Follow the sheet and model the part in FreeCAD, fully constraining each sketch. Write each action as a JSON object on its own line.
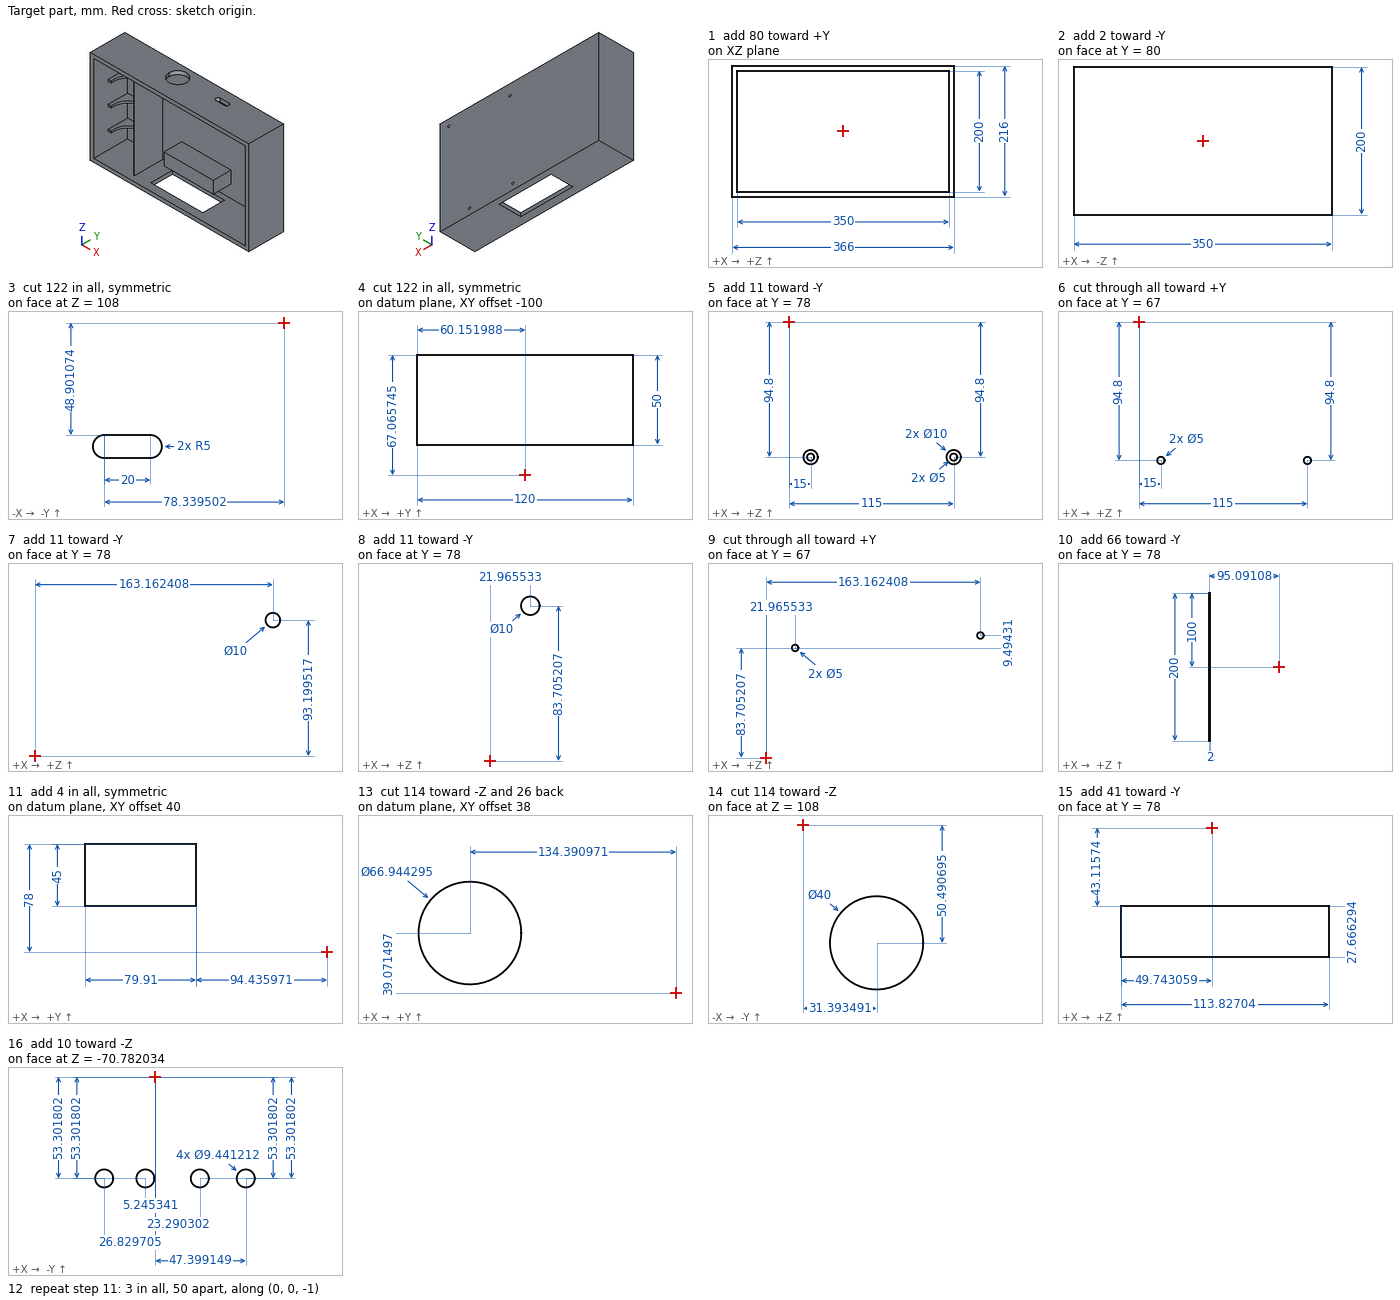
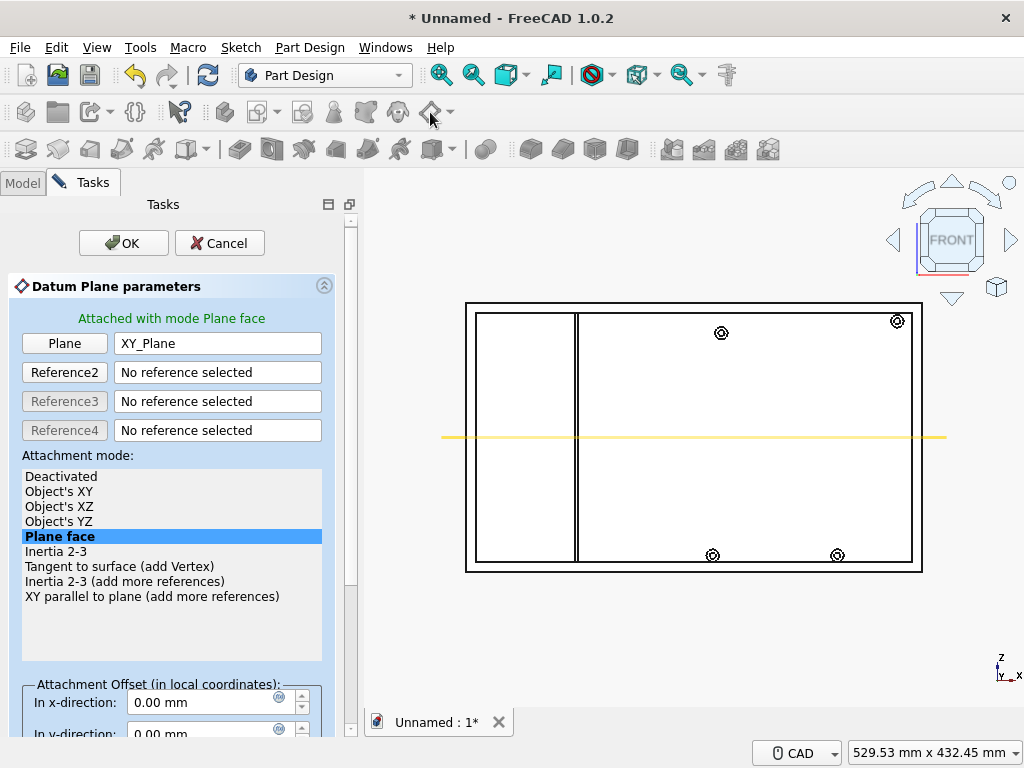
{"action": "scroll", "coordinate": [351, 475], "scroll_direction": "down", "scroll_amount": 2}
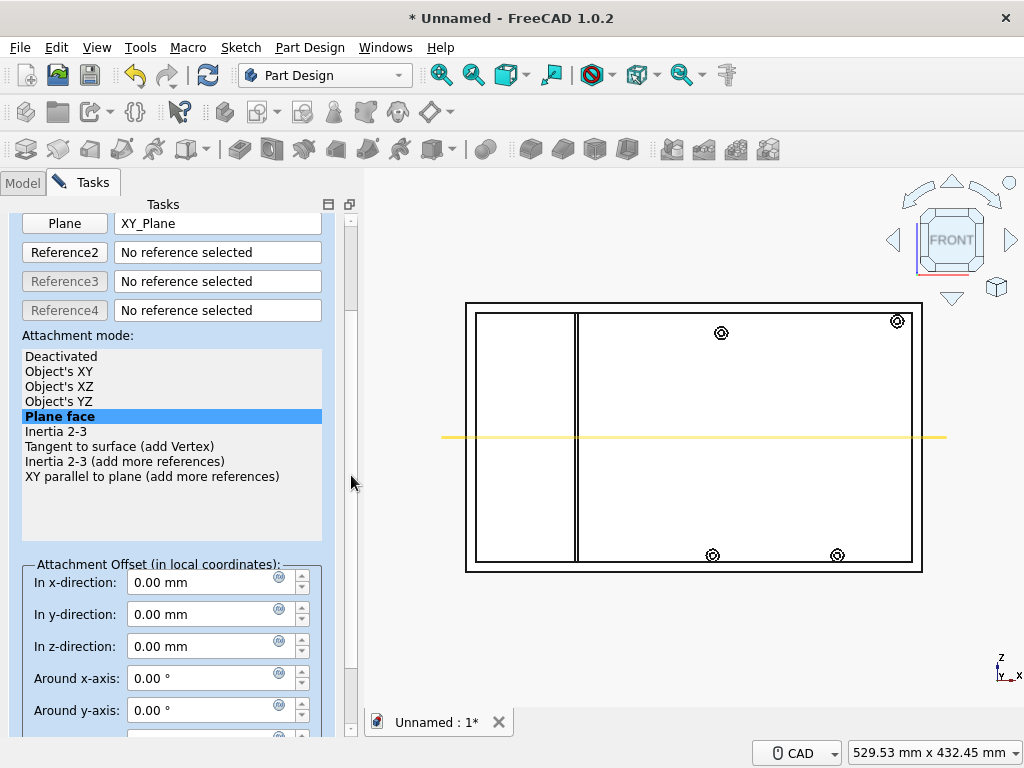
{"action": "triple_click", "coordinate": [210, 646]}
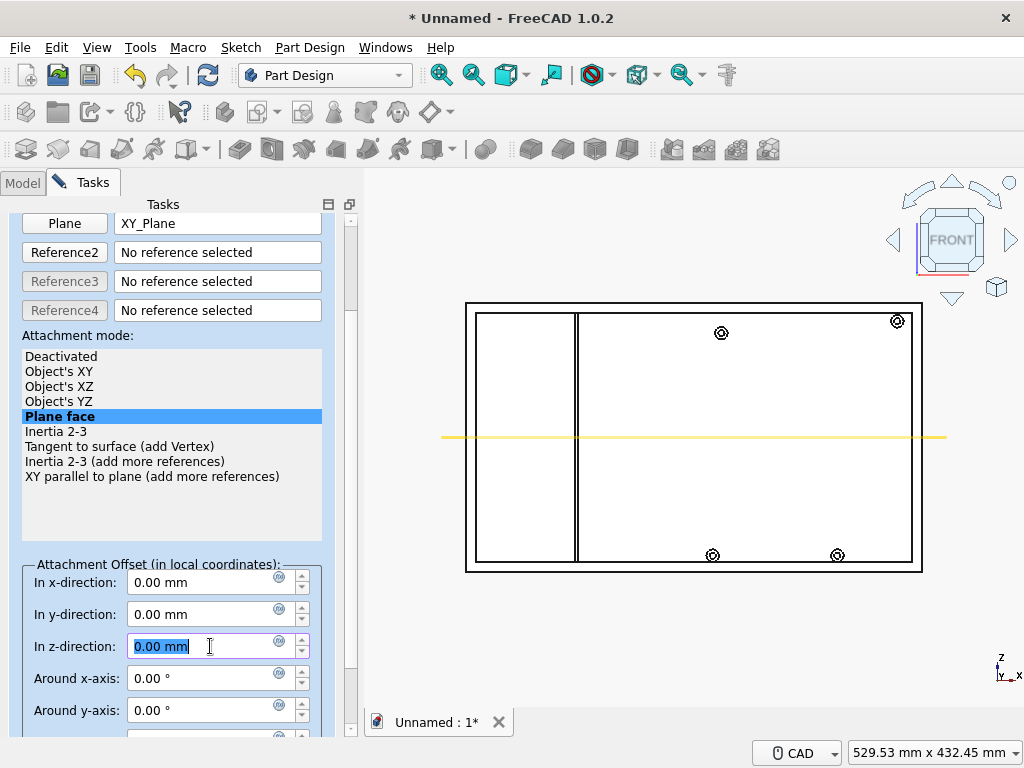
{"action": "type", "text": "40"}
{"action": "key", "text": "Tab"}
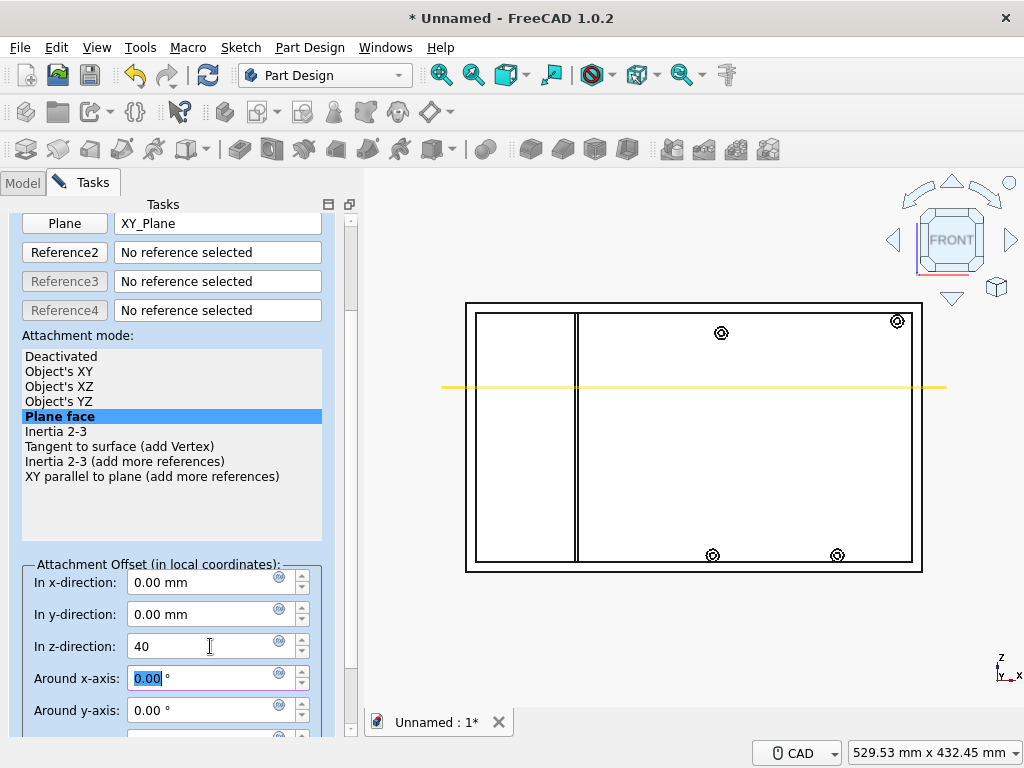
{"action": "scroll", "coordinate": [351, 475], "scroll_direction": "up", "scroll_amount": 3}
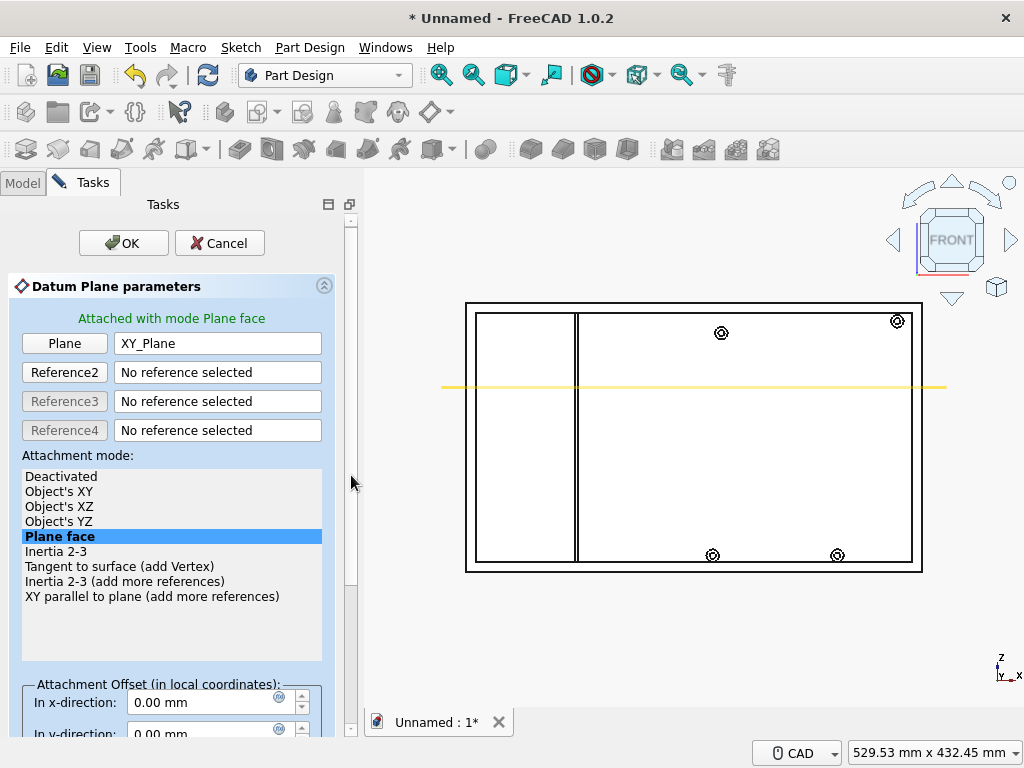
{"action": "left_click", "coordinate": [124, 243]}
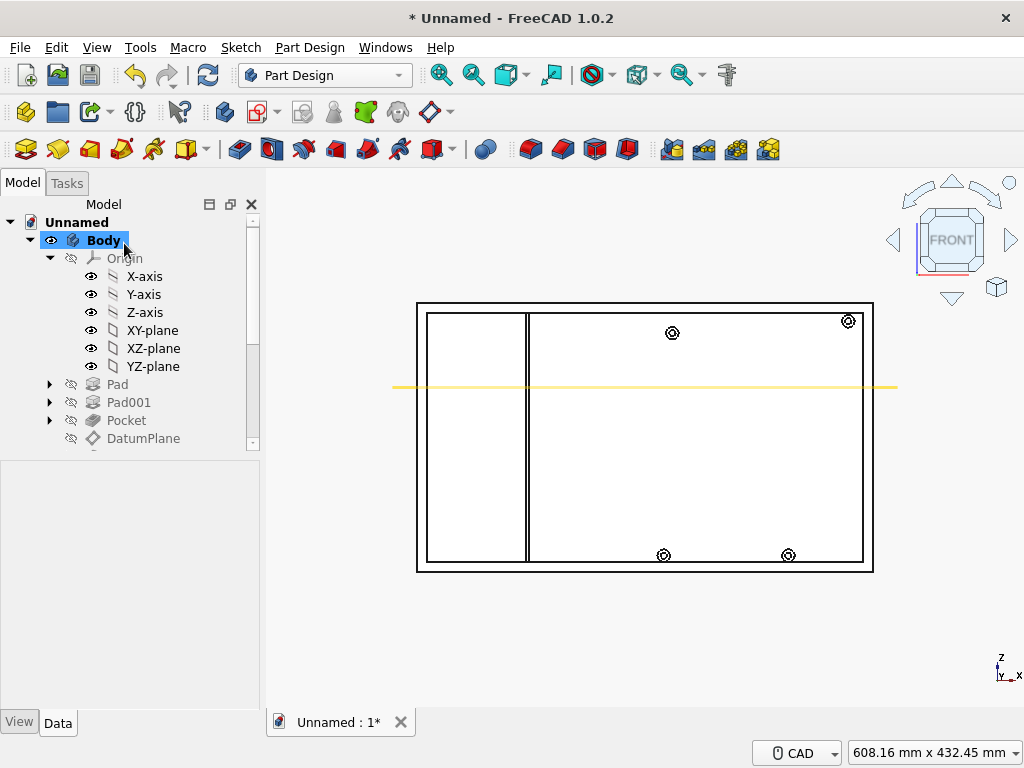
{"action": "scroll", "coordinate": [100, 326], "scroll_direction": "down", "scroll_amount": 3}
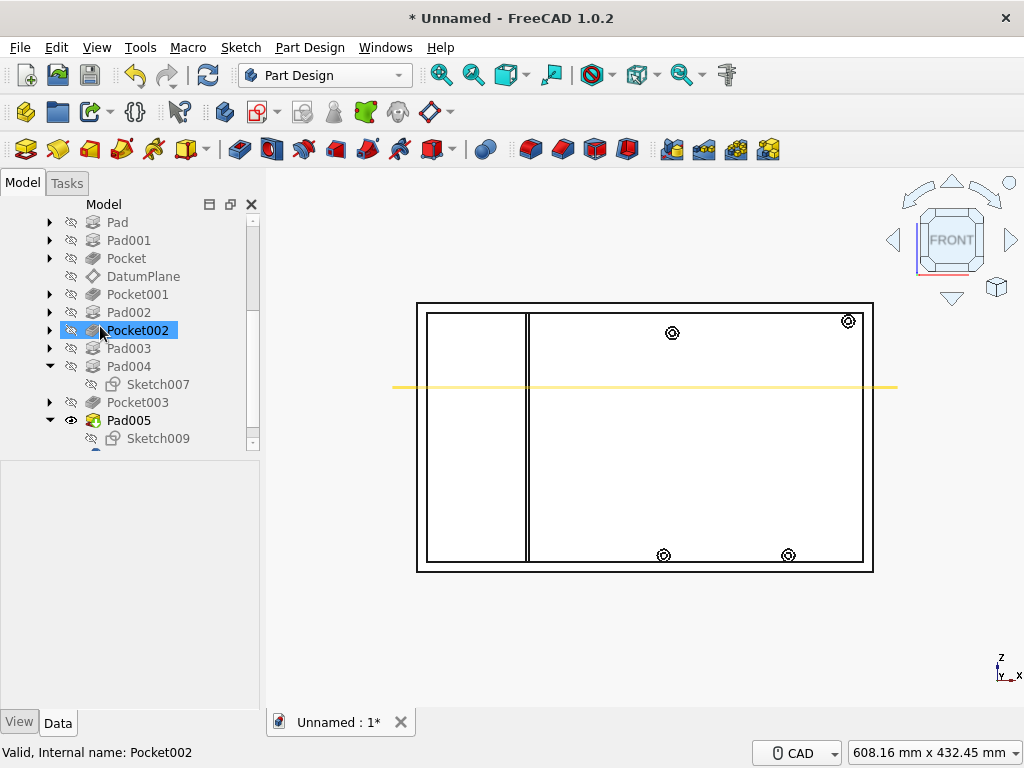
{"action": "scroll", "coordinate": [140, 326], "scroll_direction": "up", "scroll_amount": 15}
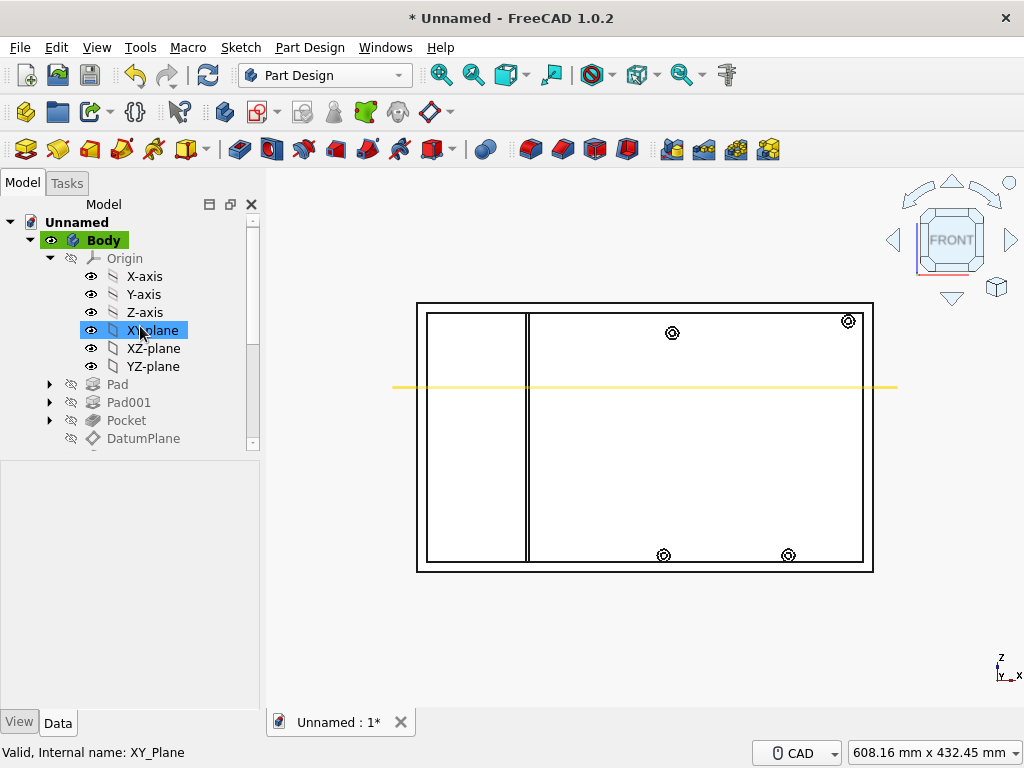
{"action": "scroll", "coordinate": [100, 326], "scroll_direction": "down", "scroll_amount": 6}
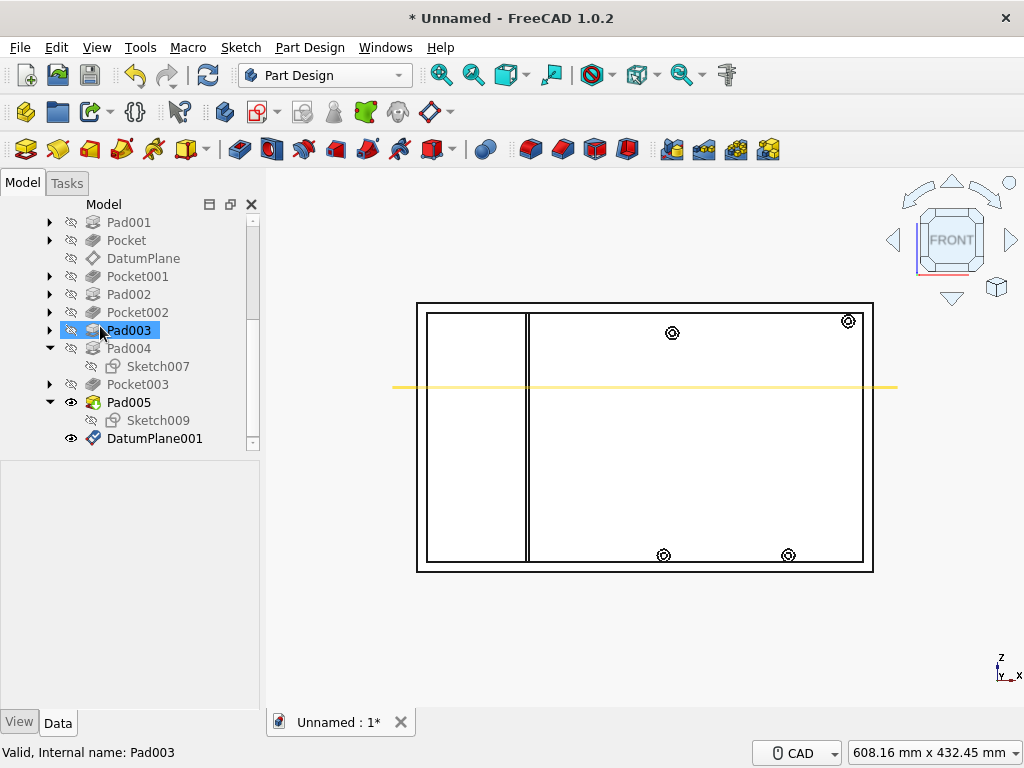
{"action": "left_click", "coordinate": [116, 438]}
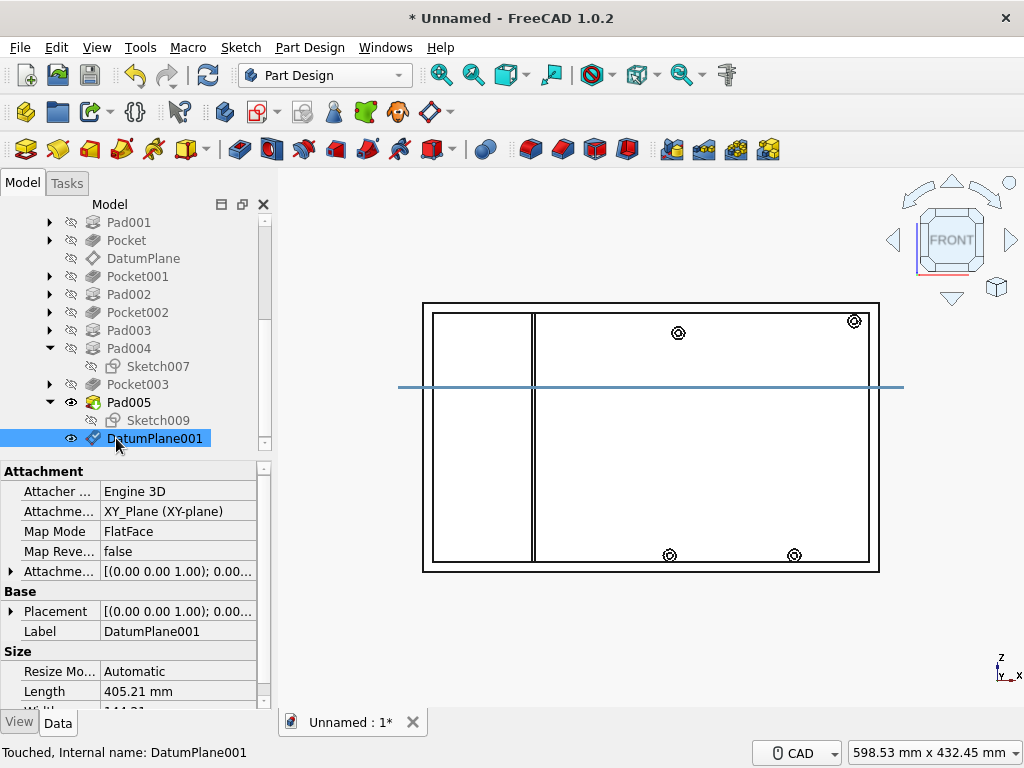
{"action": "left_click", "coordinate": [258, 112]}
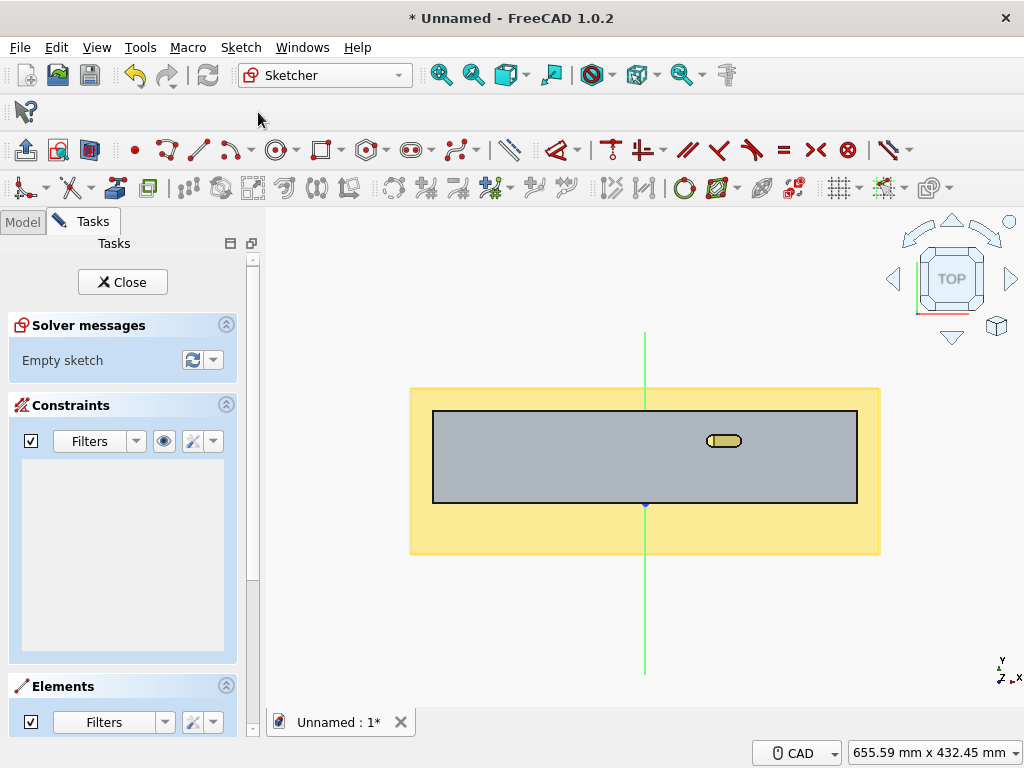
{"action": "left_click", "coordinate": [90, 150]}